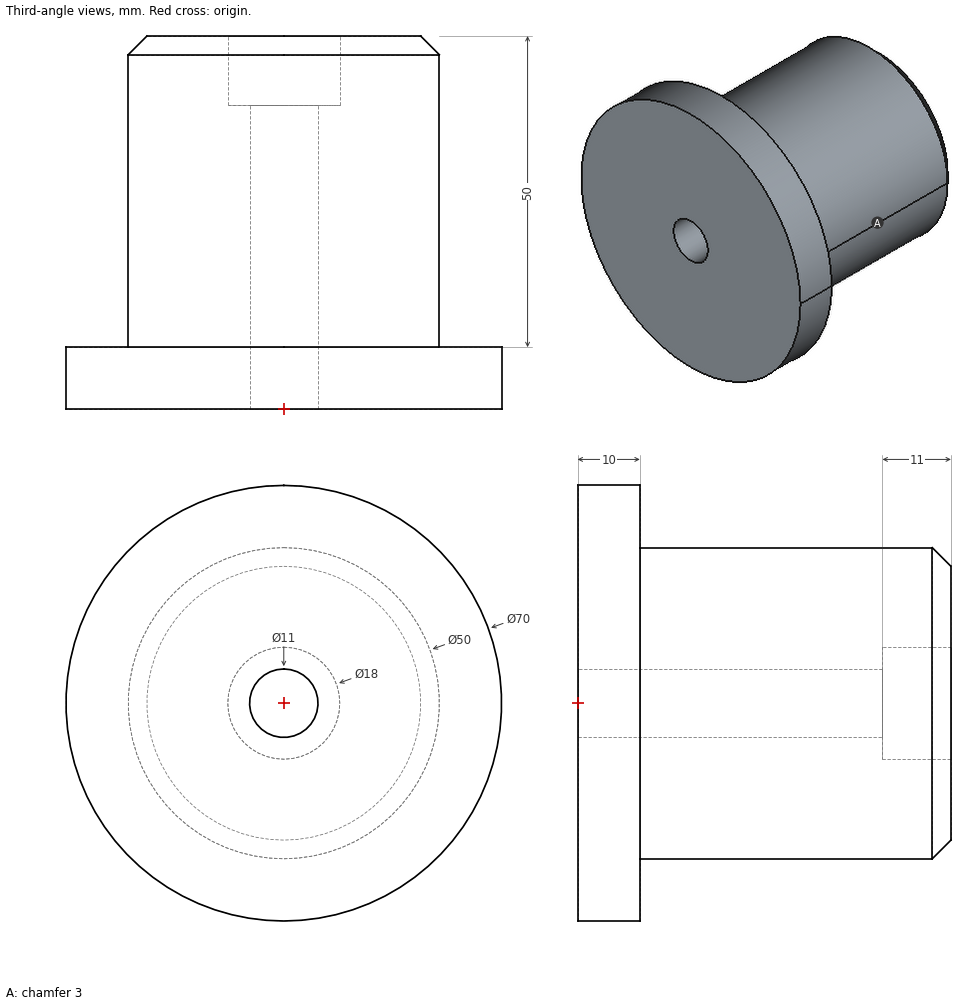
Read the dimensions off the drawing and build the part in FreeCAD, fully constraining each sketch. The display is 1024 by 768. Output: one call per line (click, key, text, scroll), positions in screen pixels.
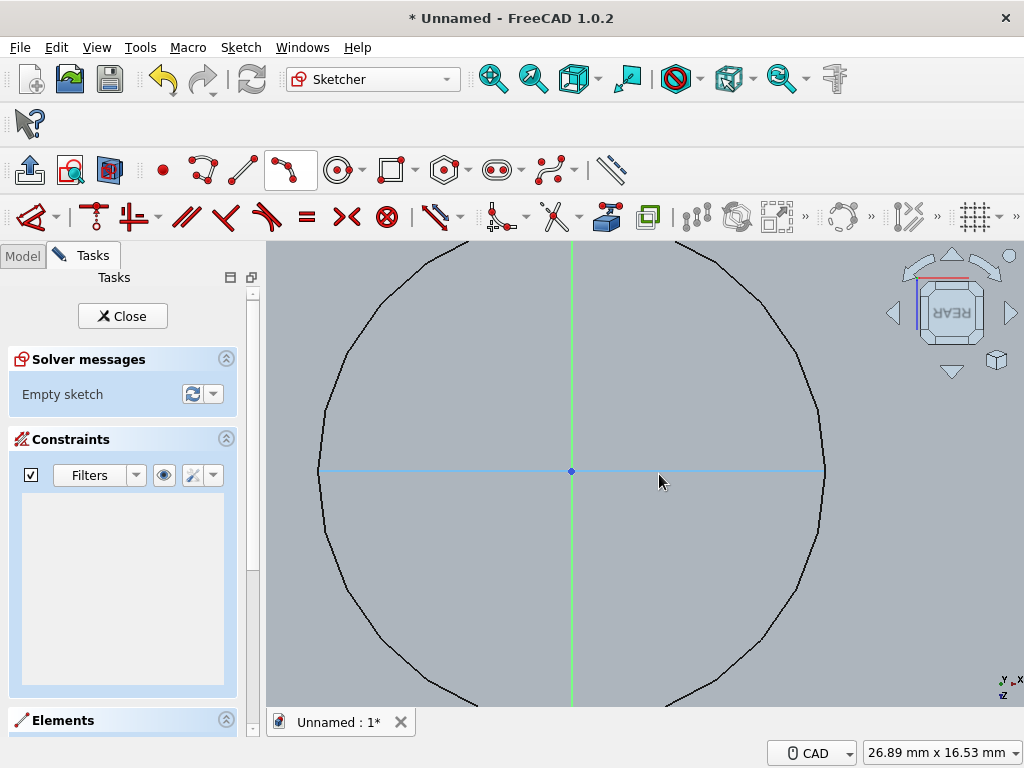
key(g)
key(c)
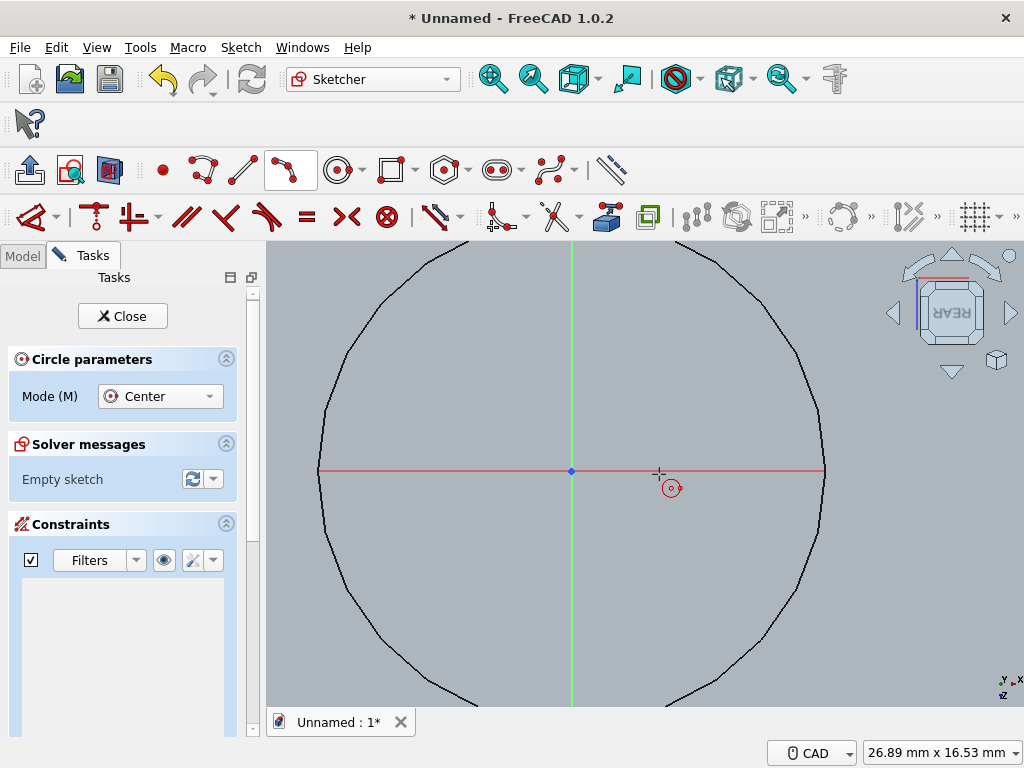
click(572, 471)
move(681, 362)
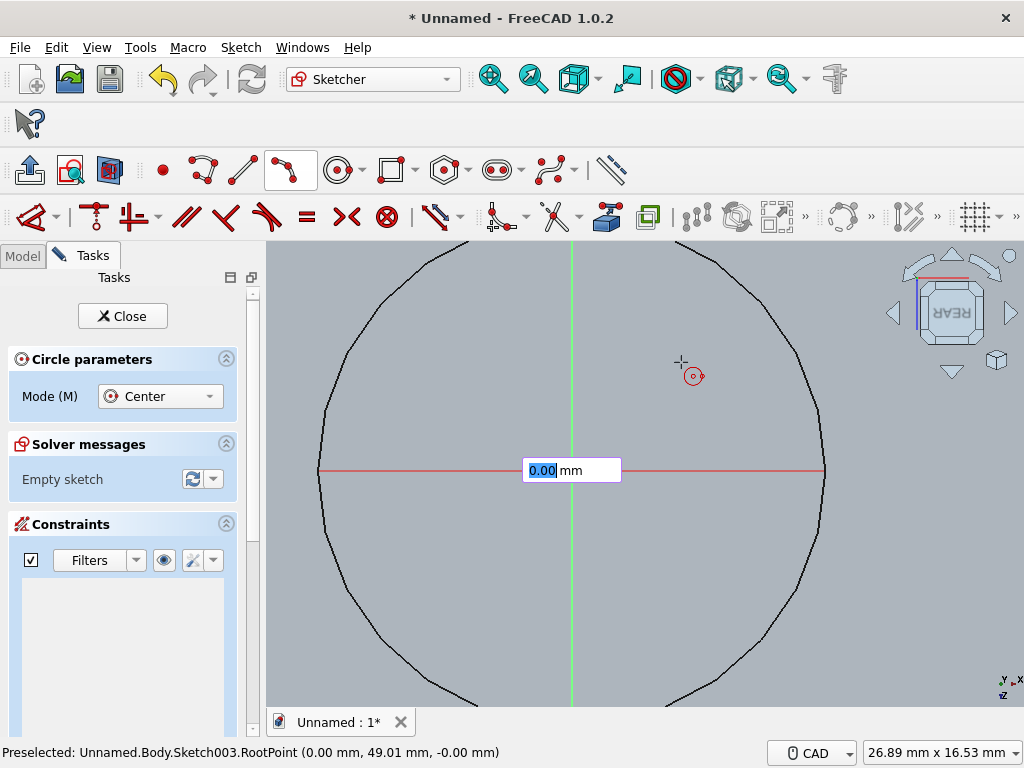
text(11)
key(Return)
key(Escape)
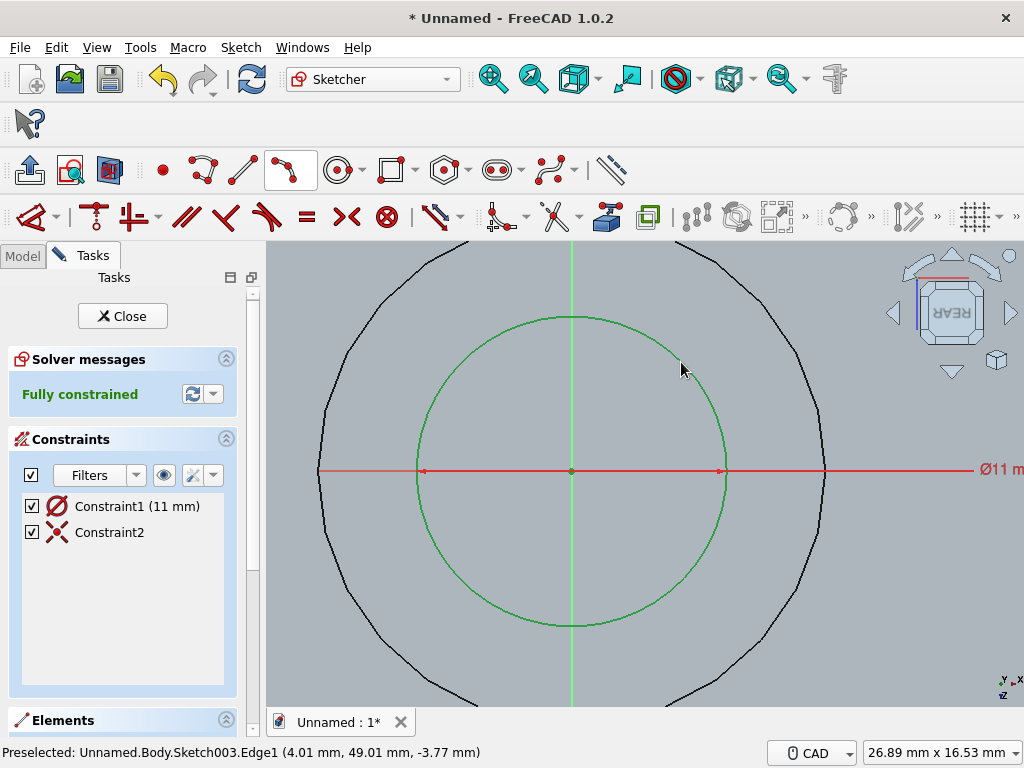
click(123, 316)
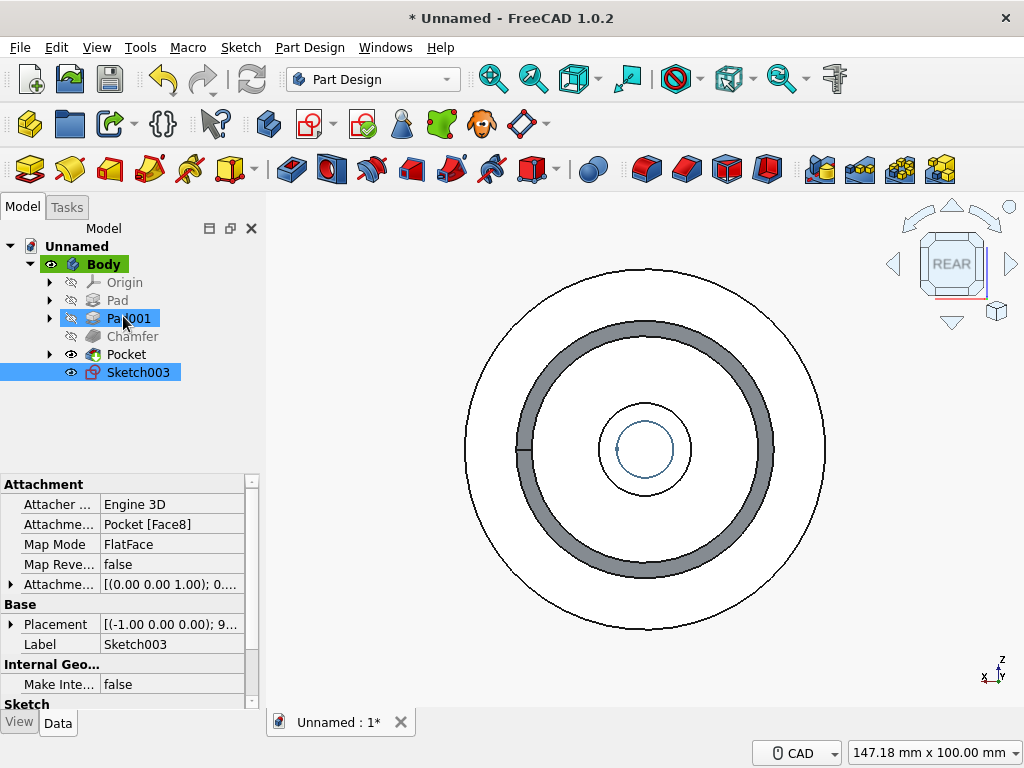
click(292, 170)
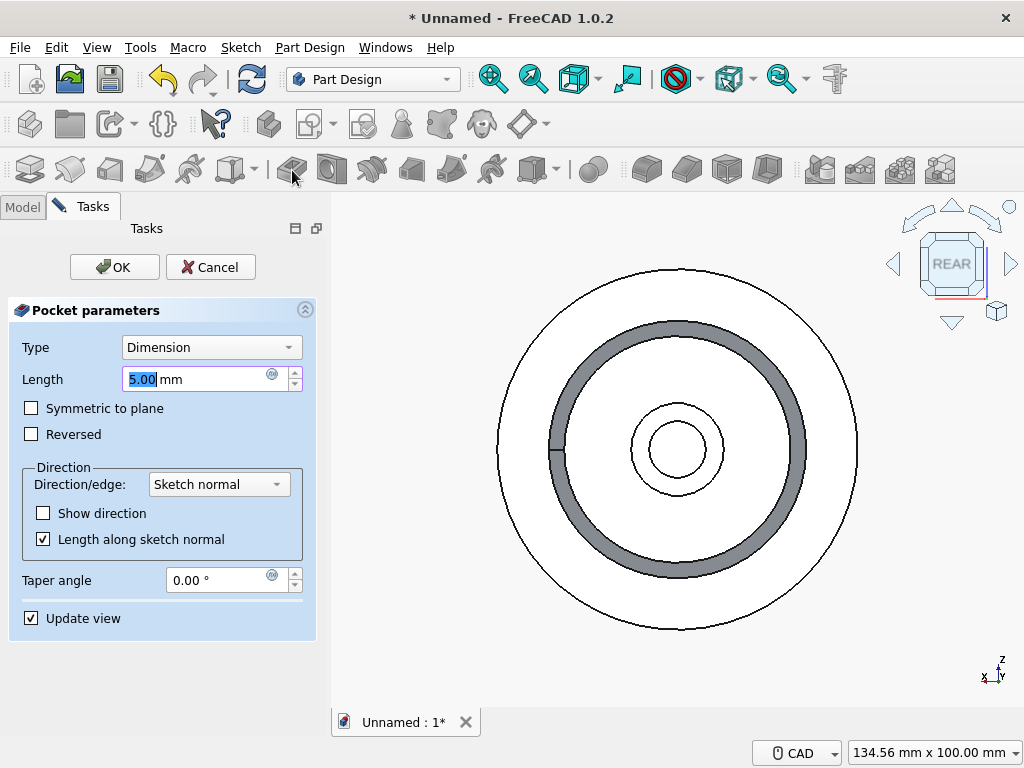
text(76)
key(Tab)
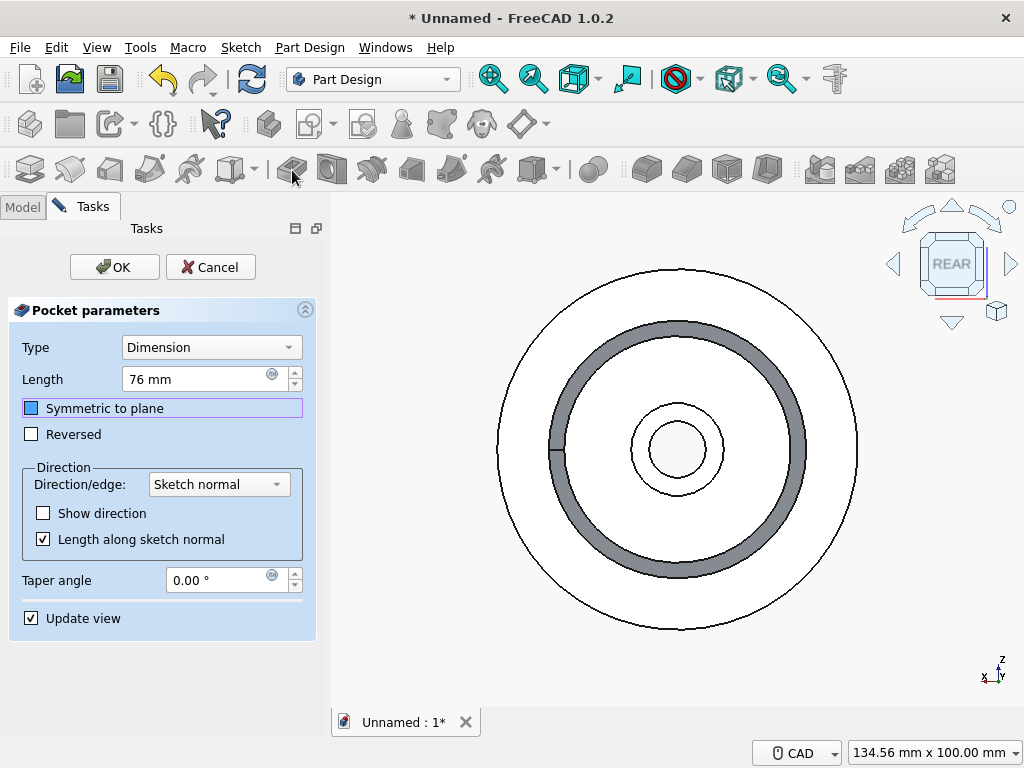
click(115, 267)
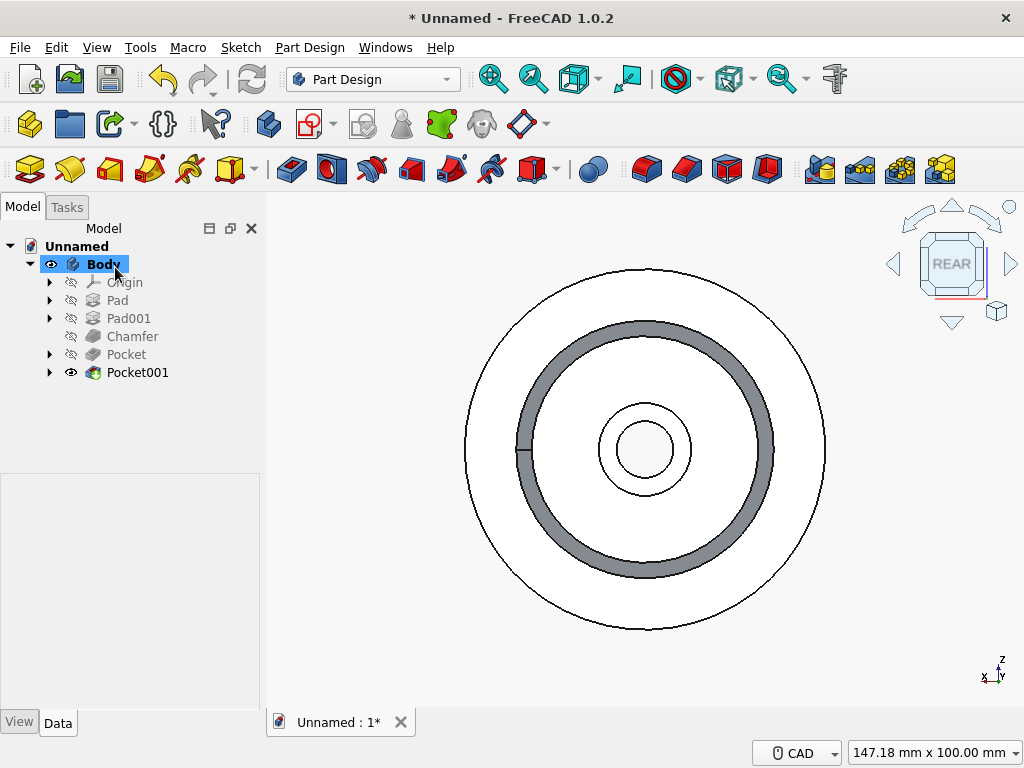
key(0)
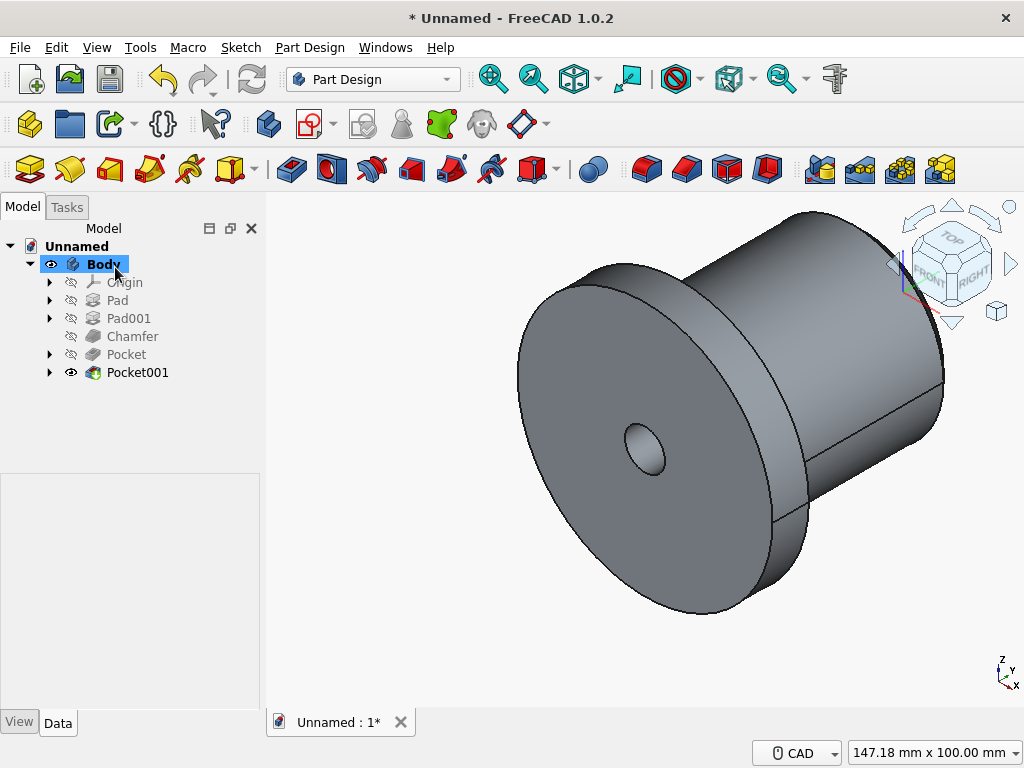
key(v)
key(f)